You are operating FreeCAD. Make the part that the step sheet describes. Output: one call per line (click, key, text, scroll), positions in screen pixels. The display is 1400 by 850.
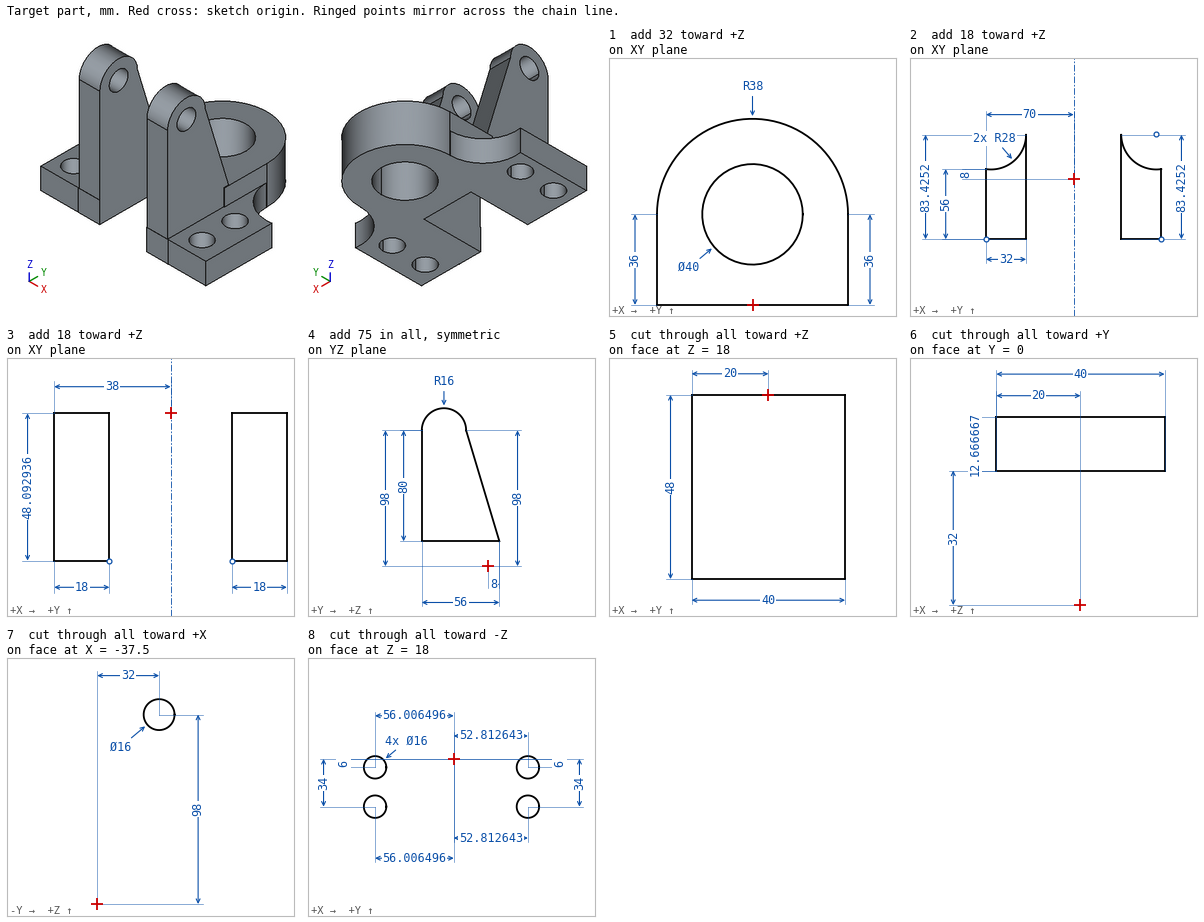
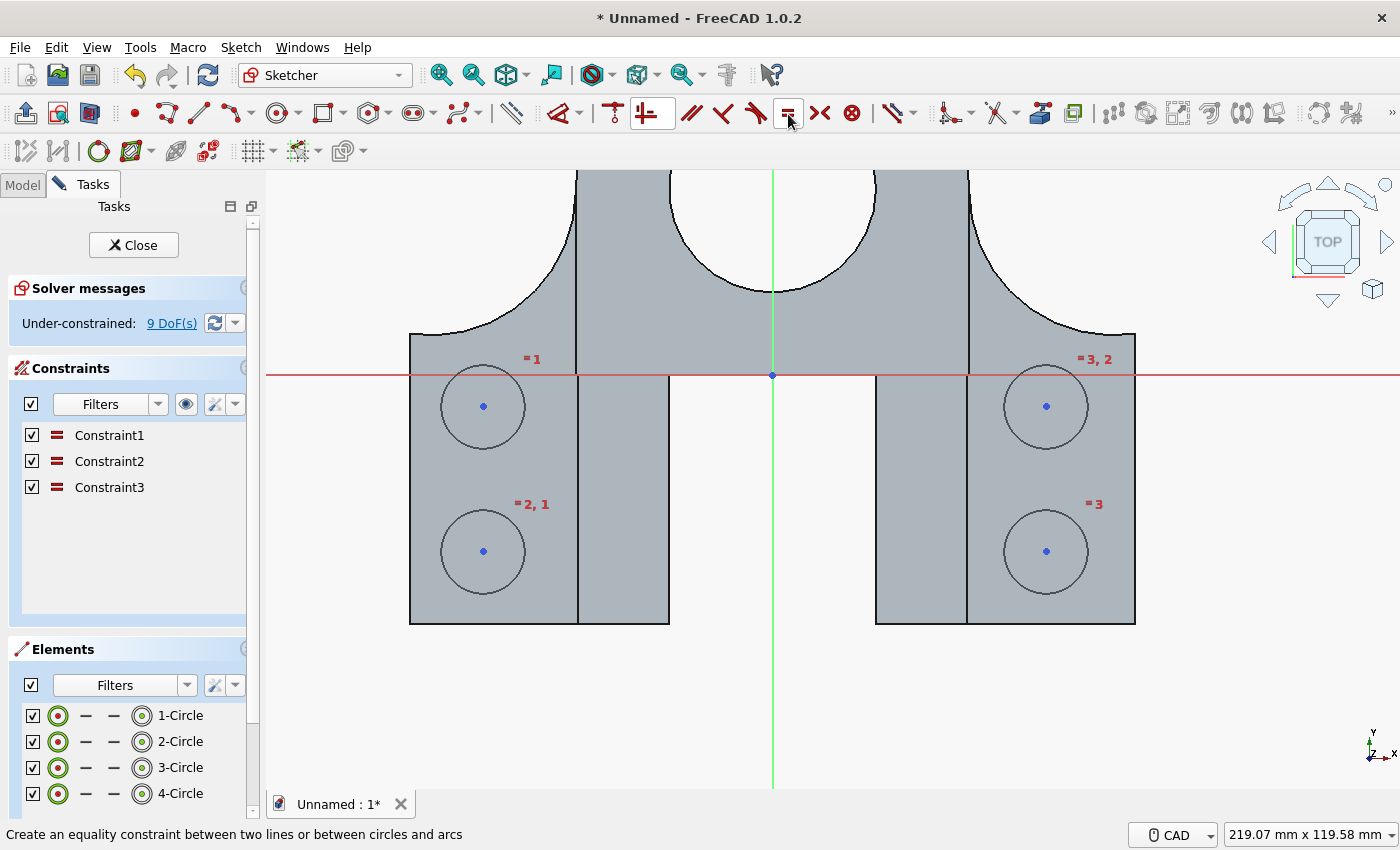
click(558, 114)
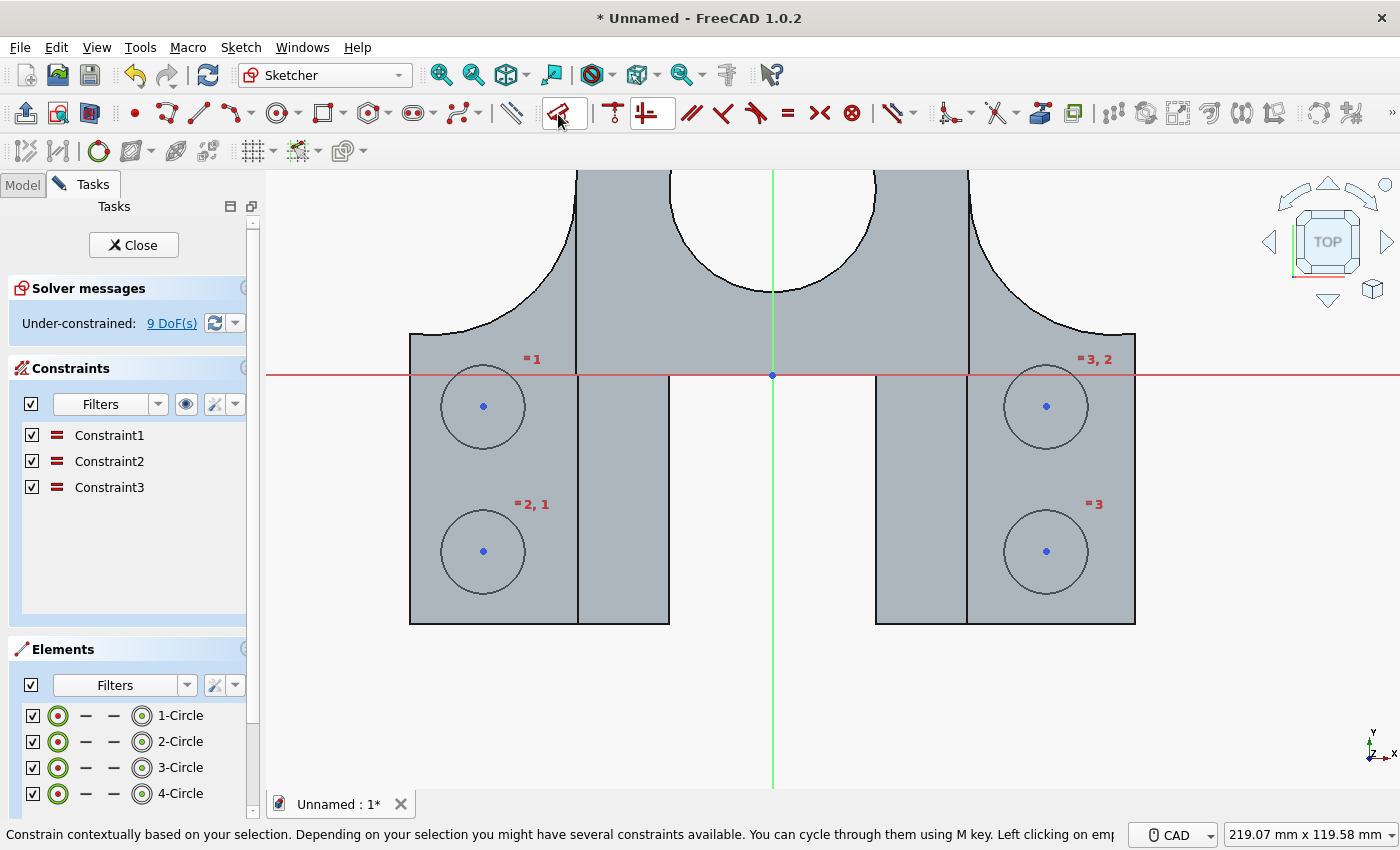
click(512, 377)
click(534, 354)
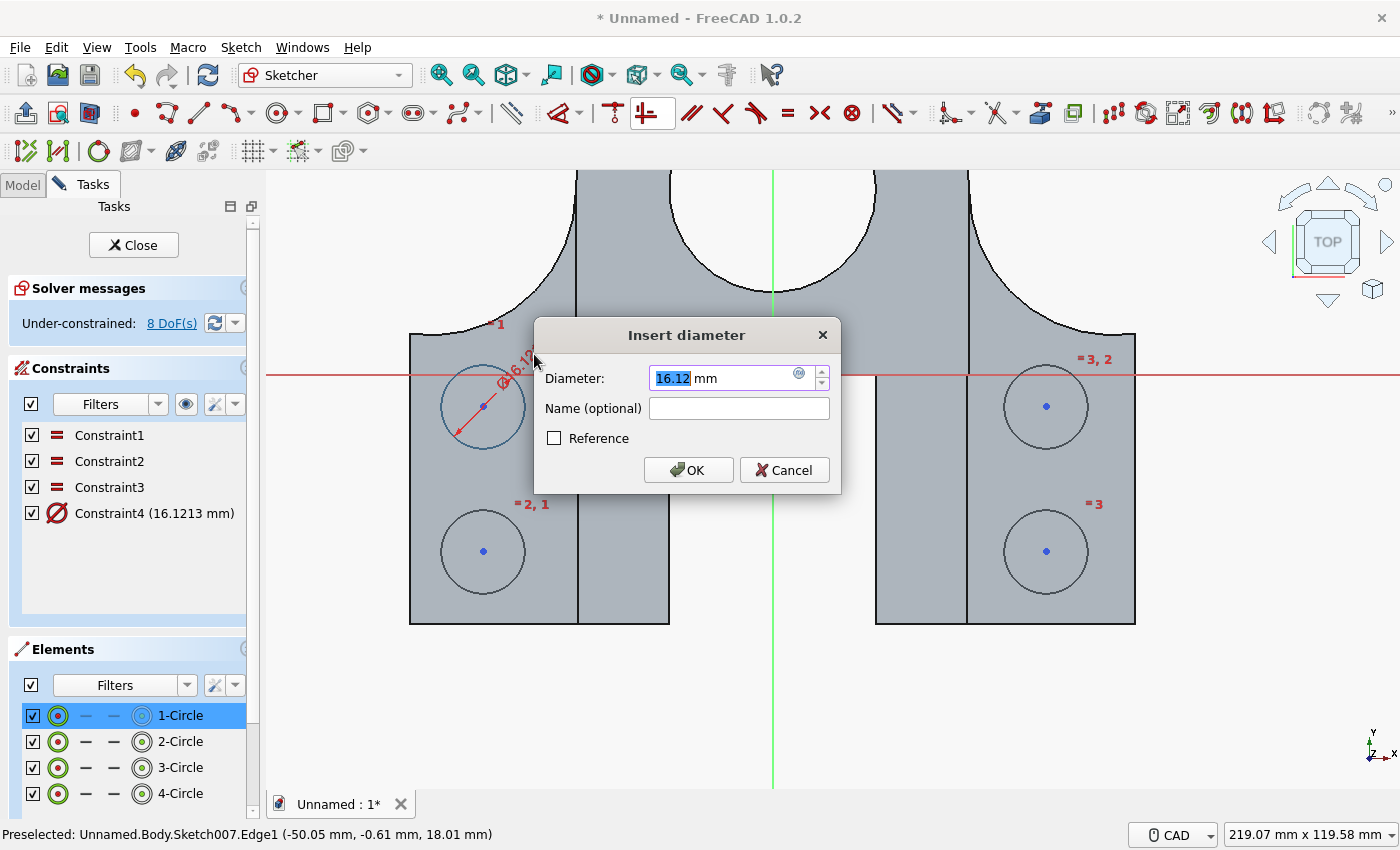
text(16)
key(Return)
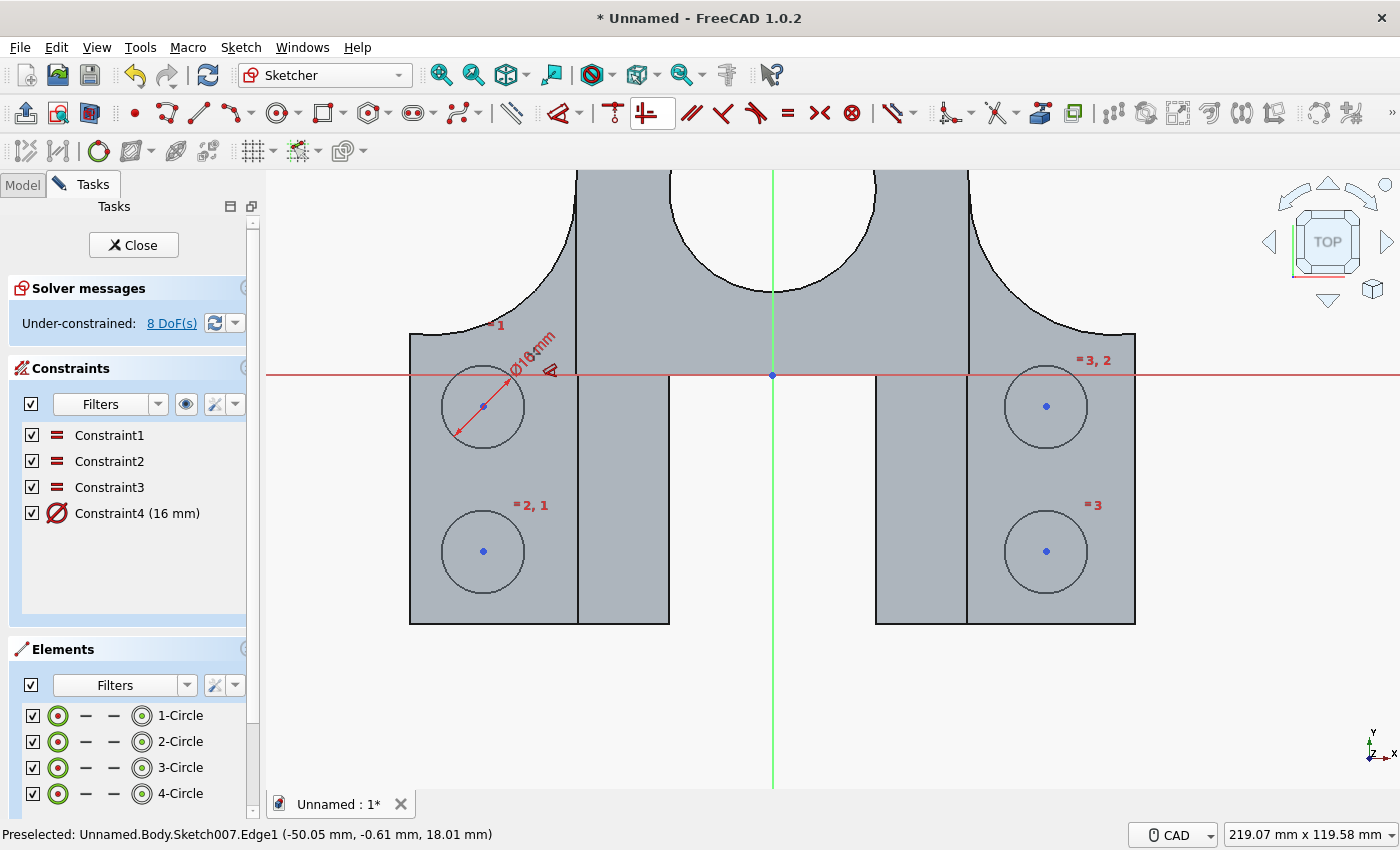
scroll(483, 407, up, 2)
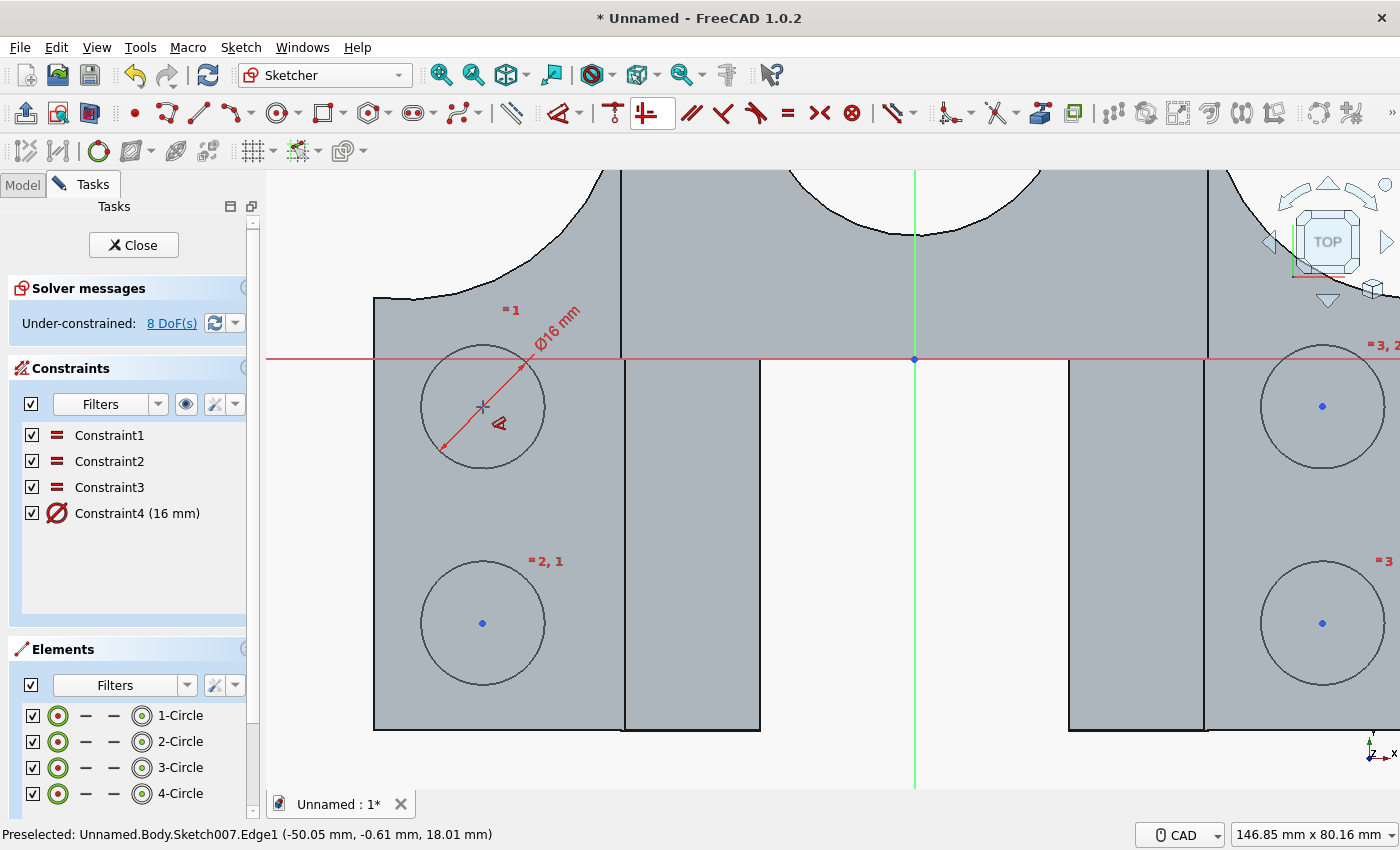
click(483, 407)
click(449, 383)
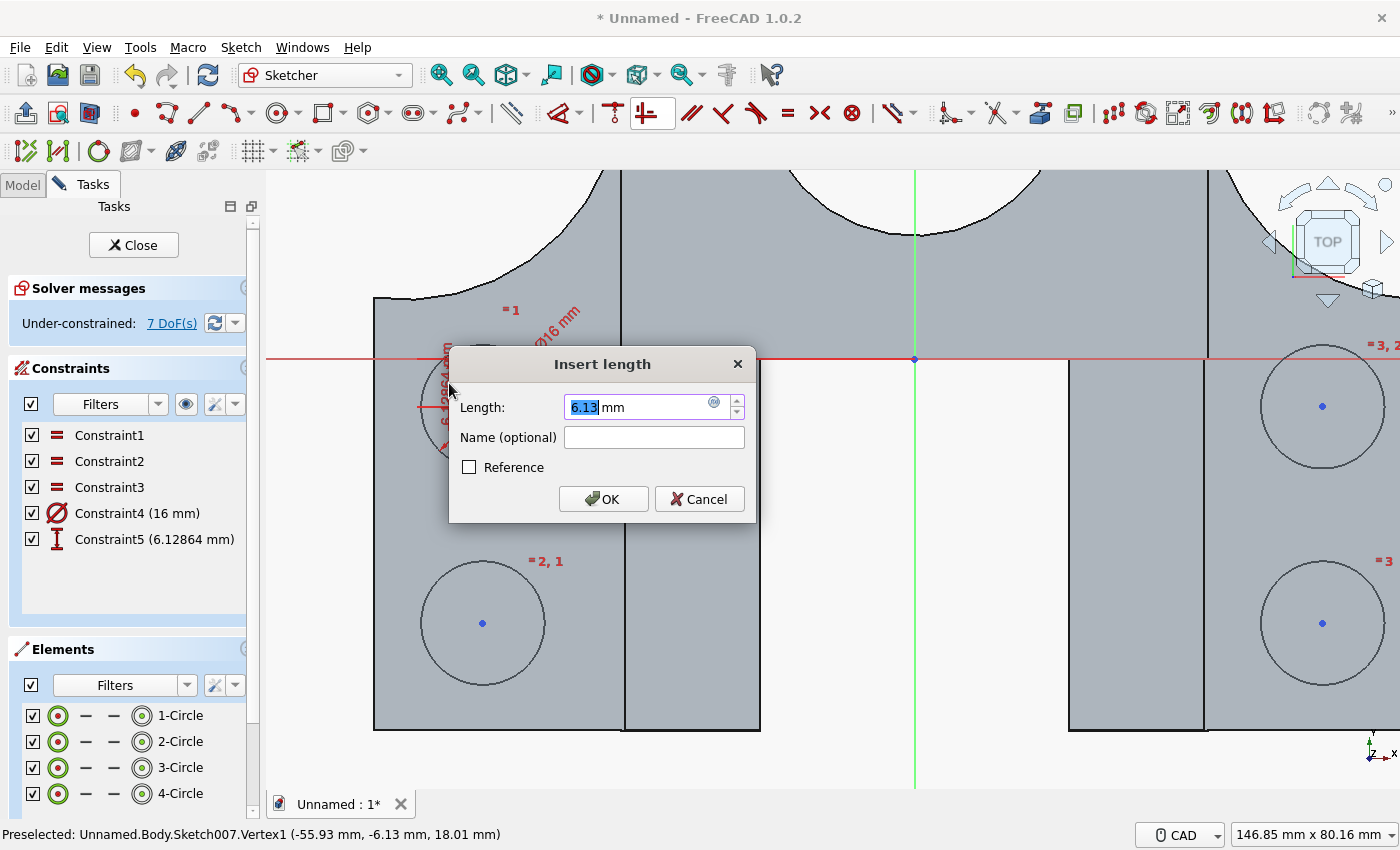
text(6)
key(Return)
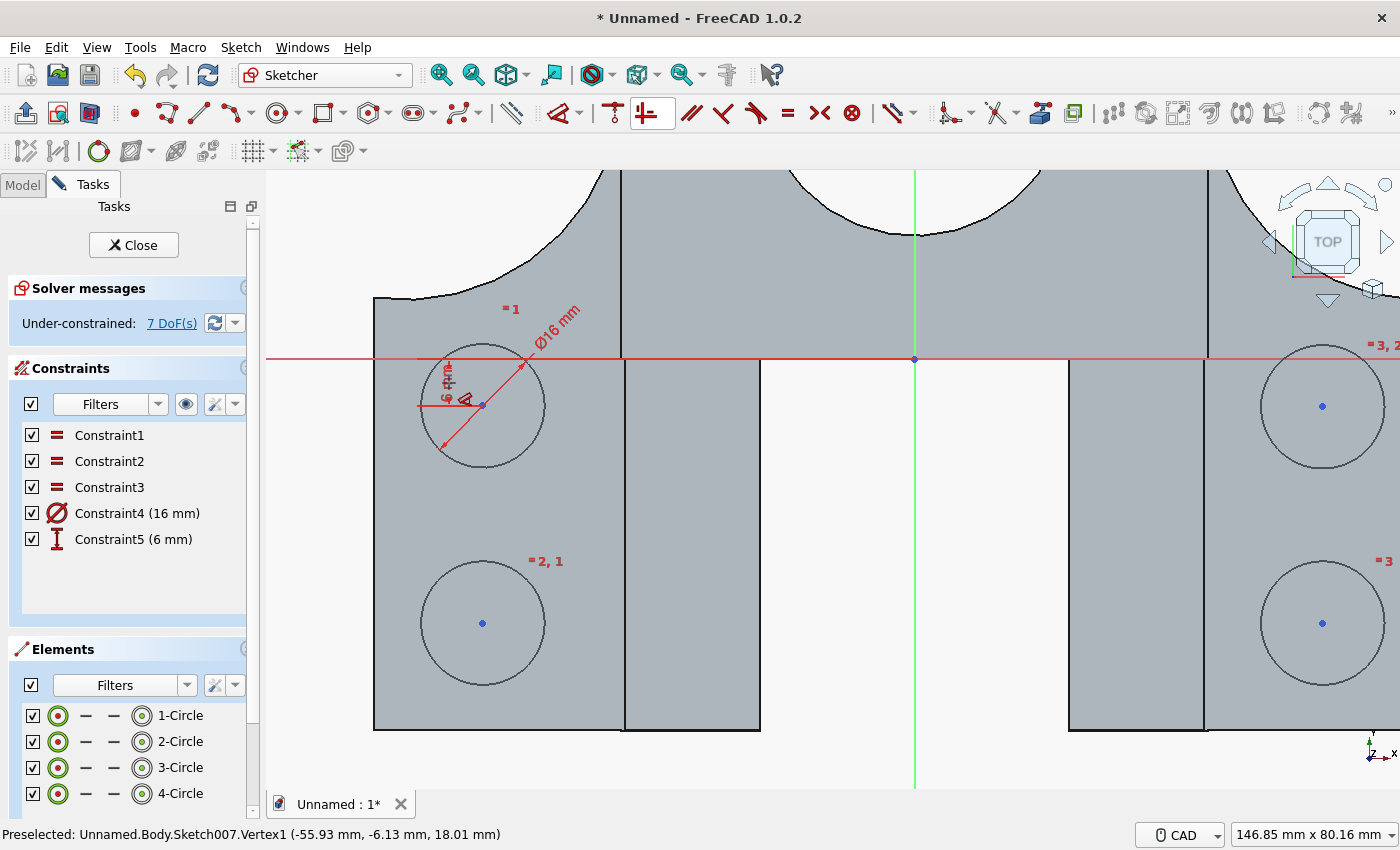
scroll(484, 409, down, 2)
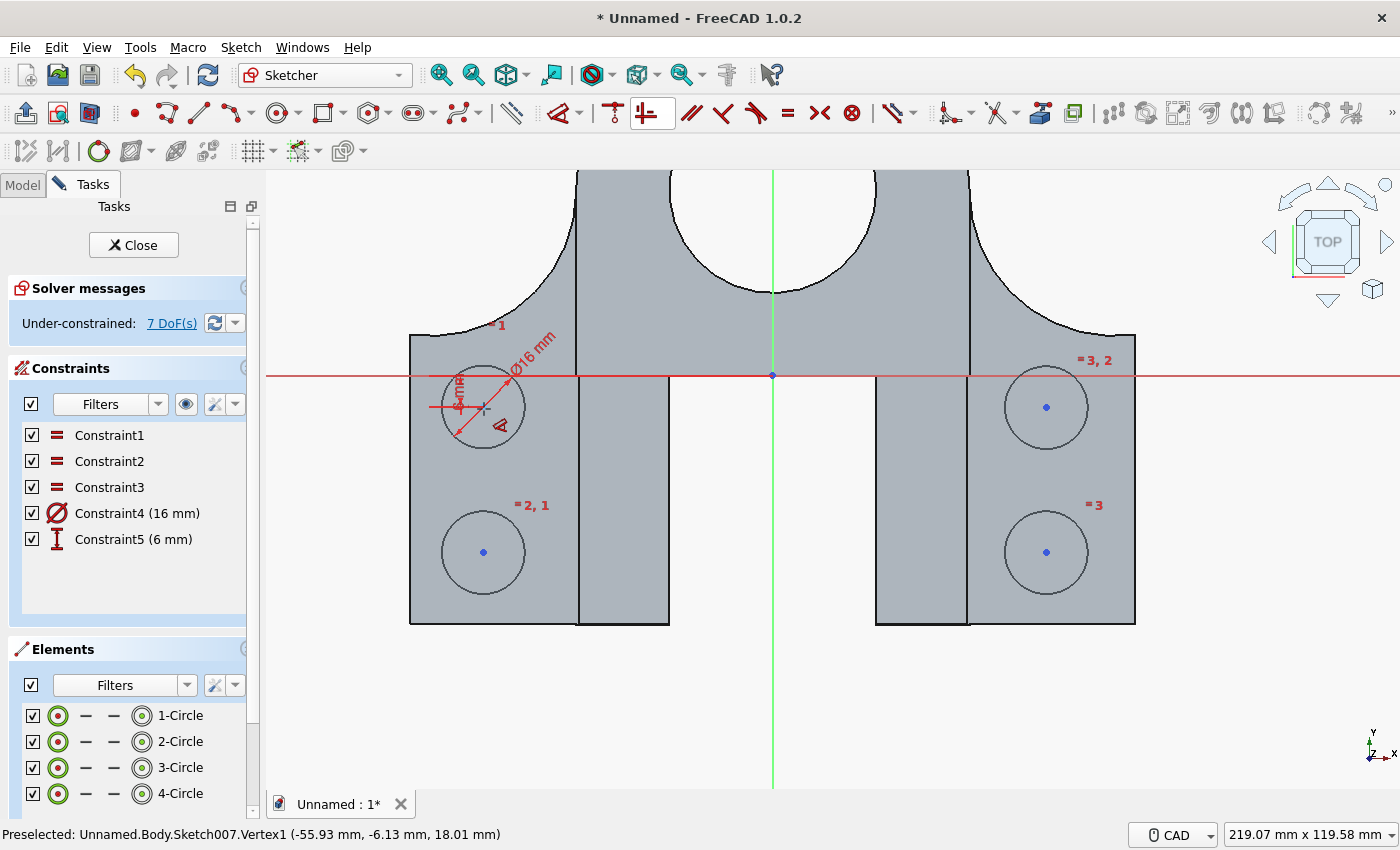
scroll(1046, 408, up, 2)